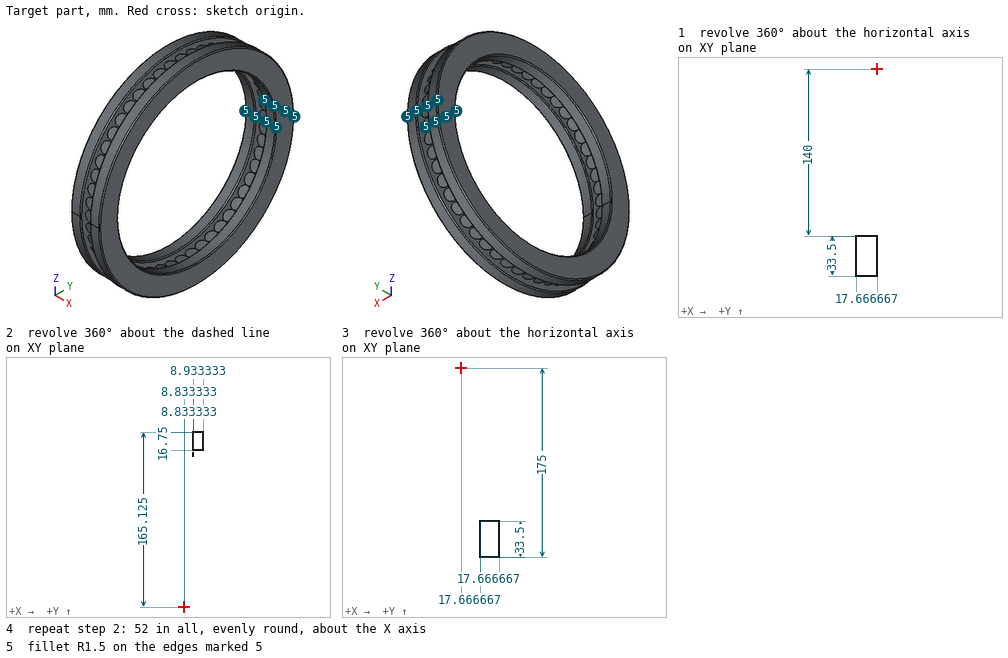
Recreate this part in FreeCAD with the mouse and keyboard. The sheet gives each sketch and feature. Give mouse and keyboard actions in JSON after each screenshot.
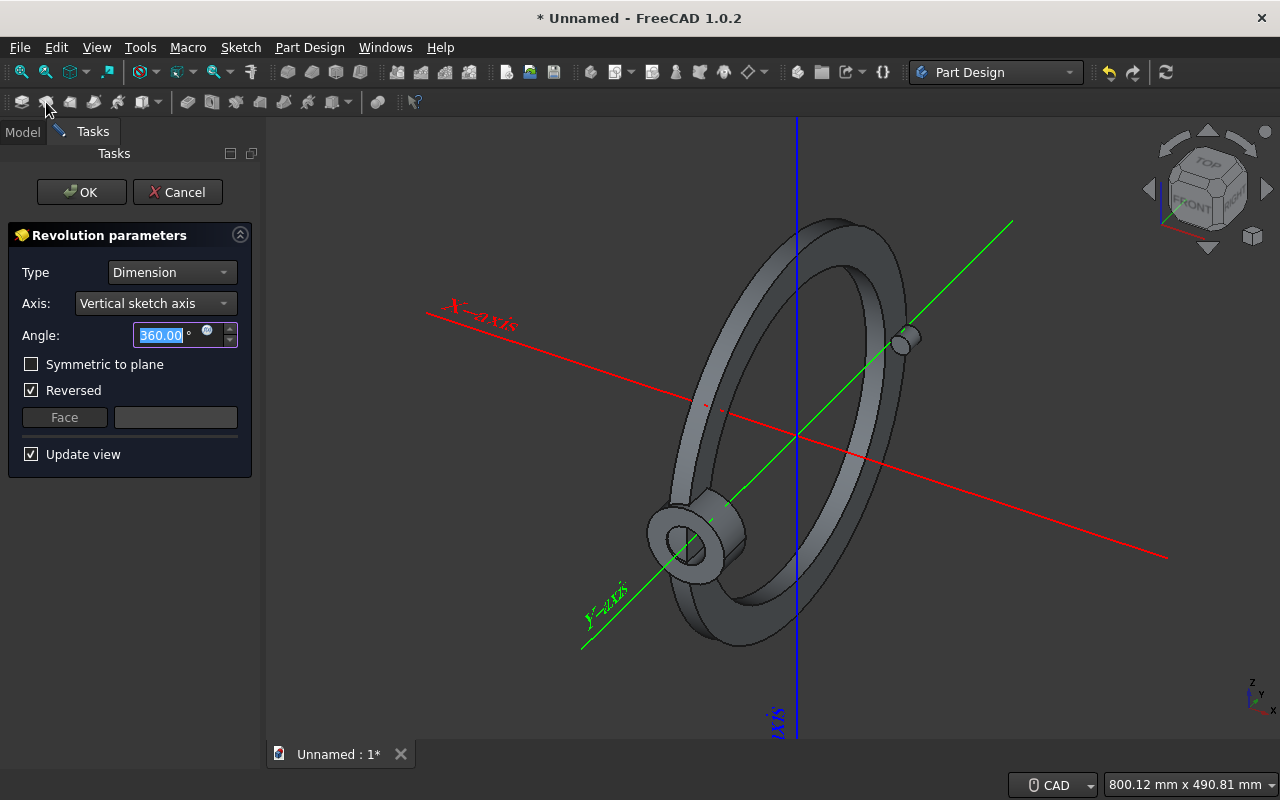
{"action": "left_click", "coordinate": [156, 304]}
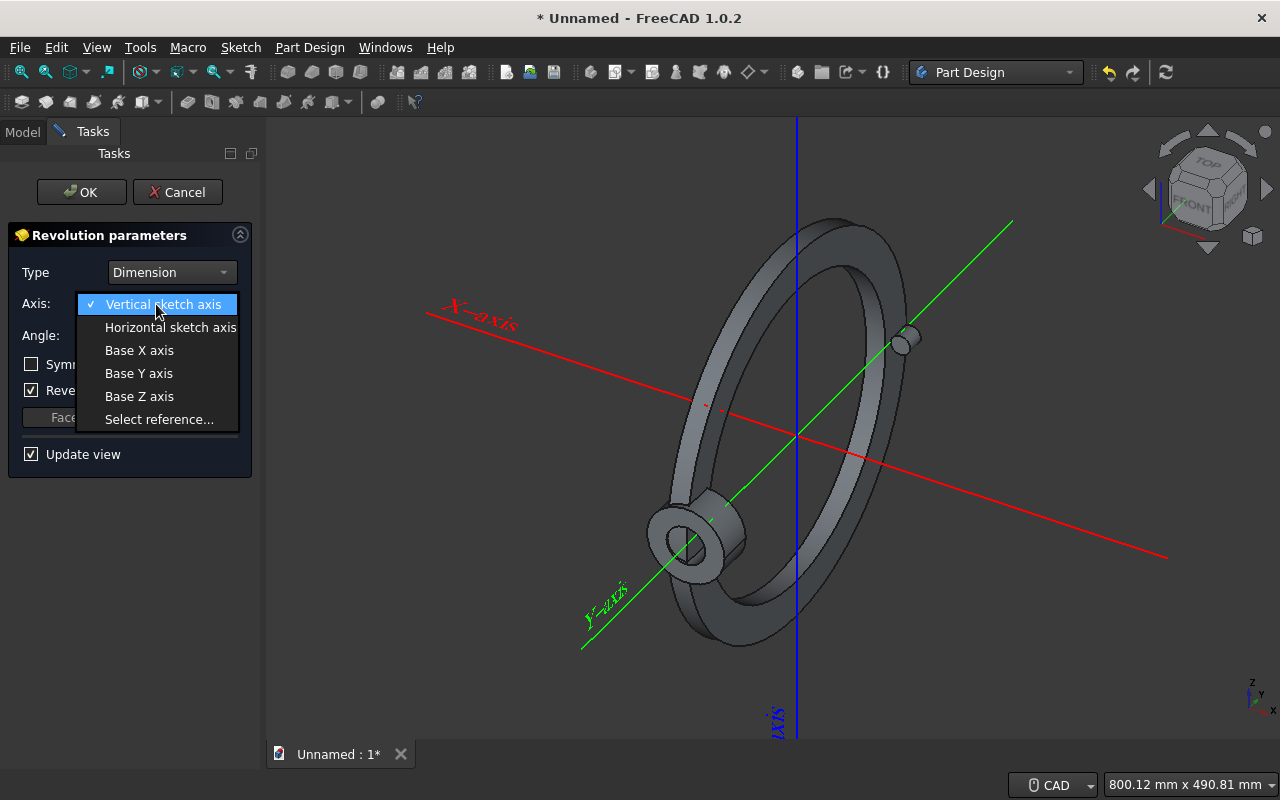
{"action": "left_click", "coordinate": [156, 328]}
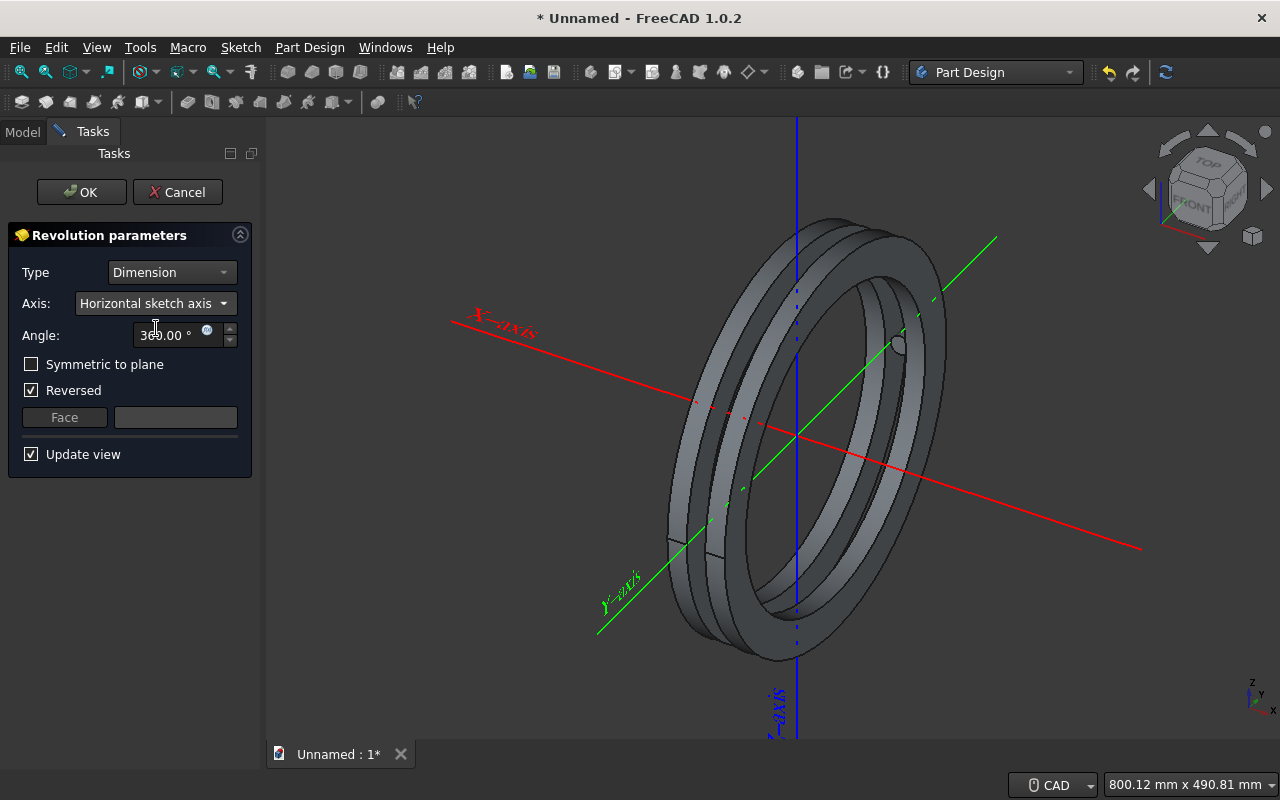
{"action": "left_click", "coordinate": [82, 192]}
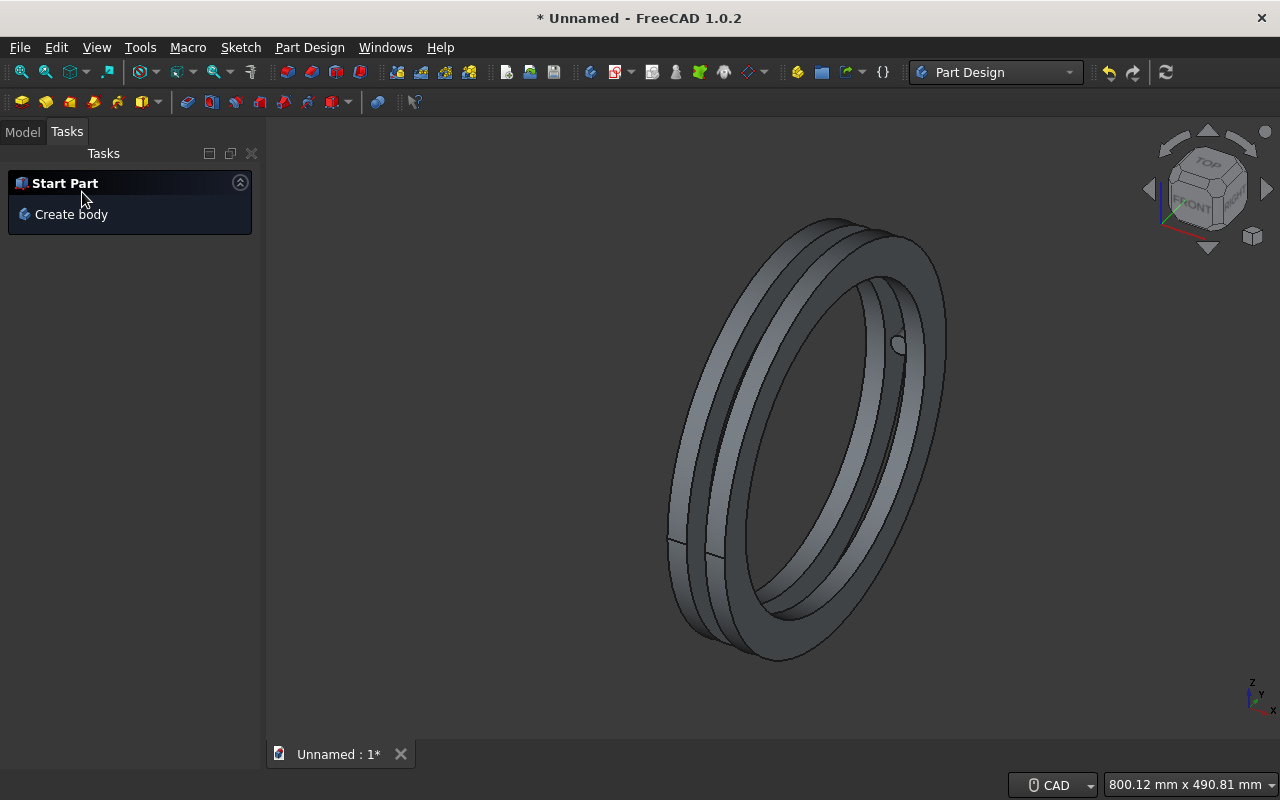
{"action": "left_click", "coordinate": [23, 131]}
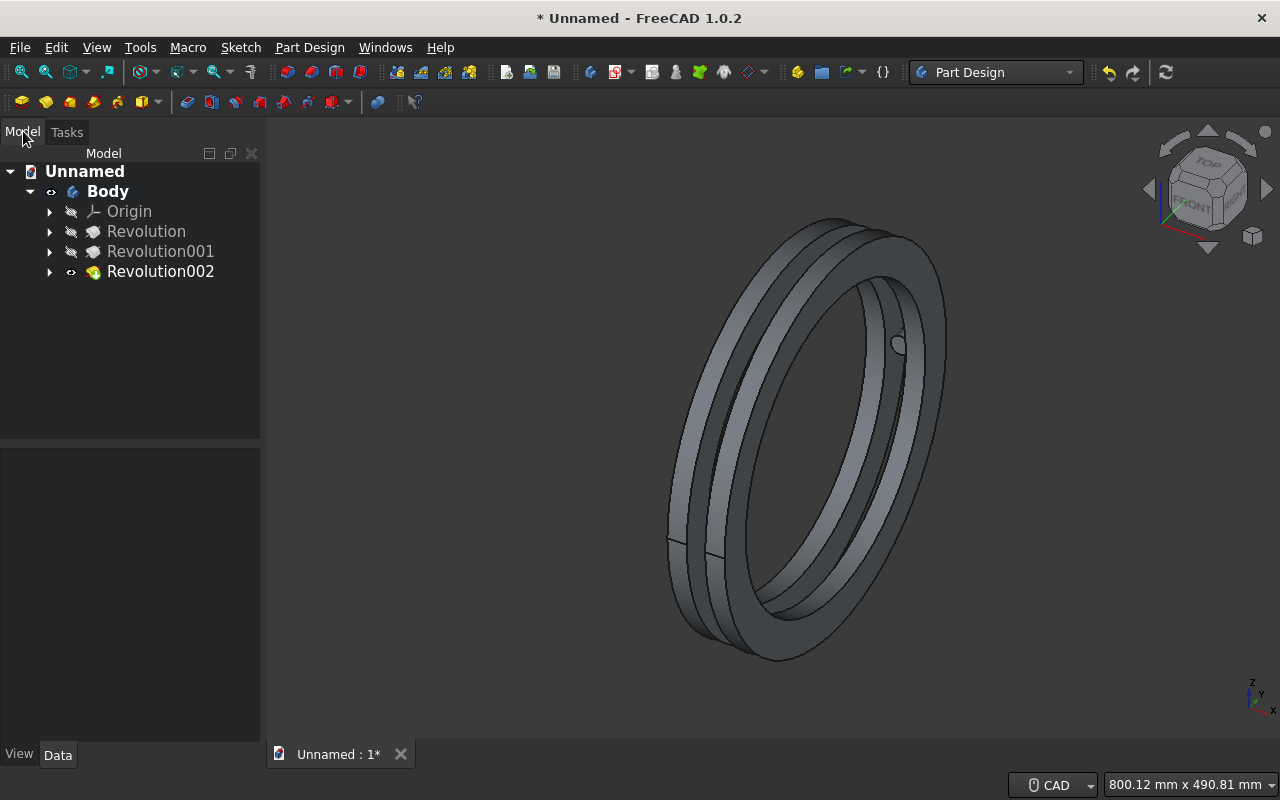
{"action": "left_click", "coordinate": [116, 252]}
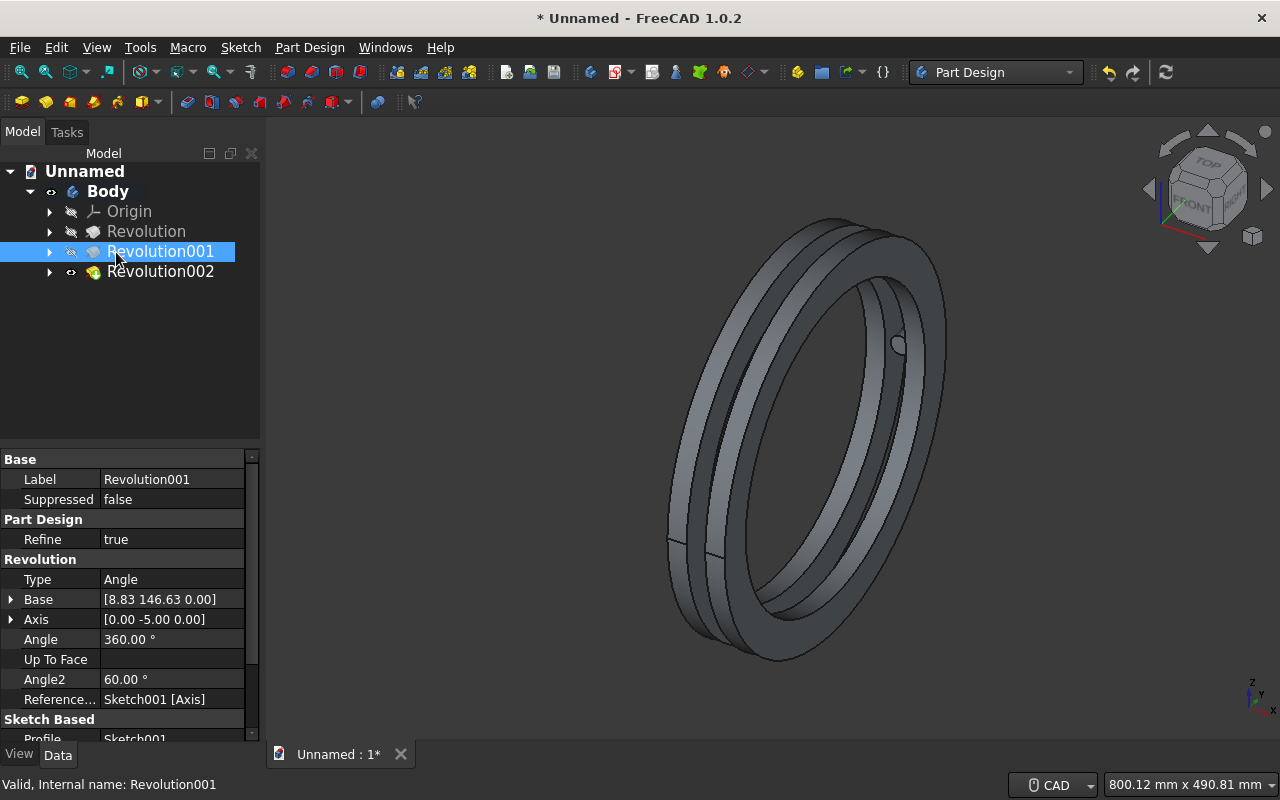
{"action": "left_click", "coordinate": [446, 72]}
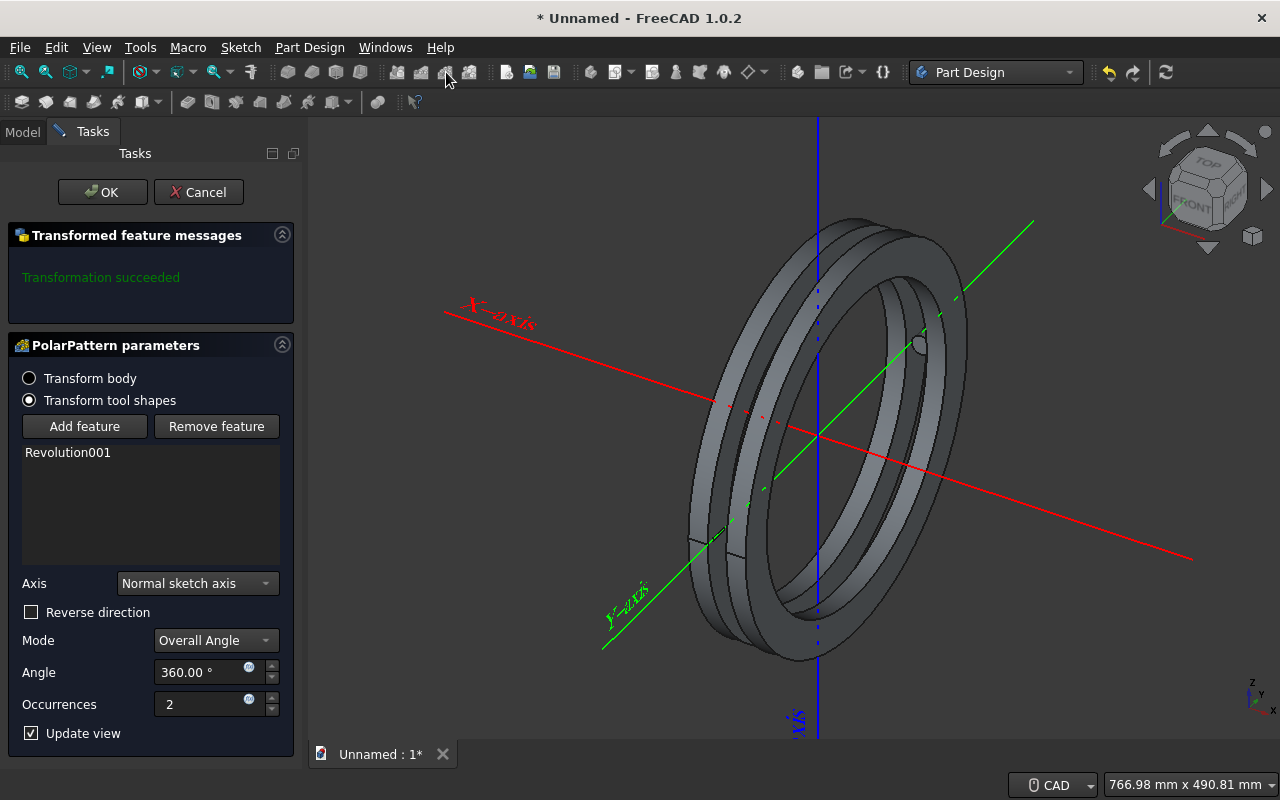
{"action": "left_click", "coordinate": [198, 584]}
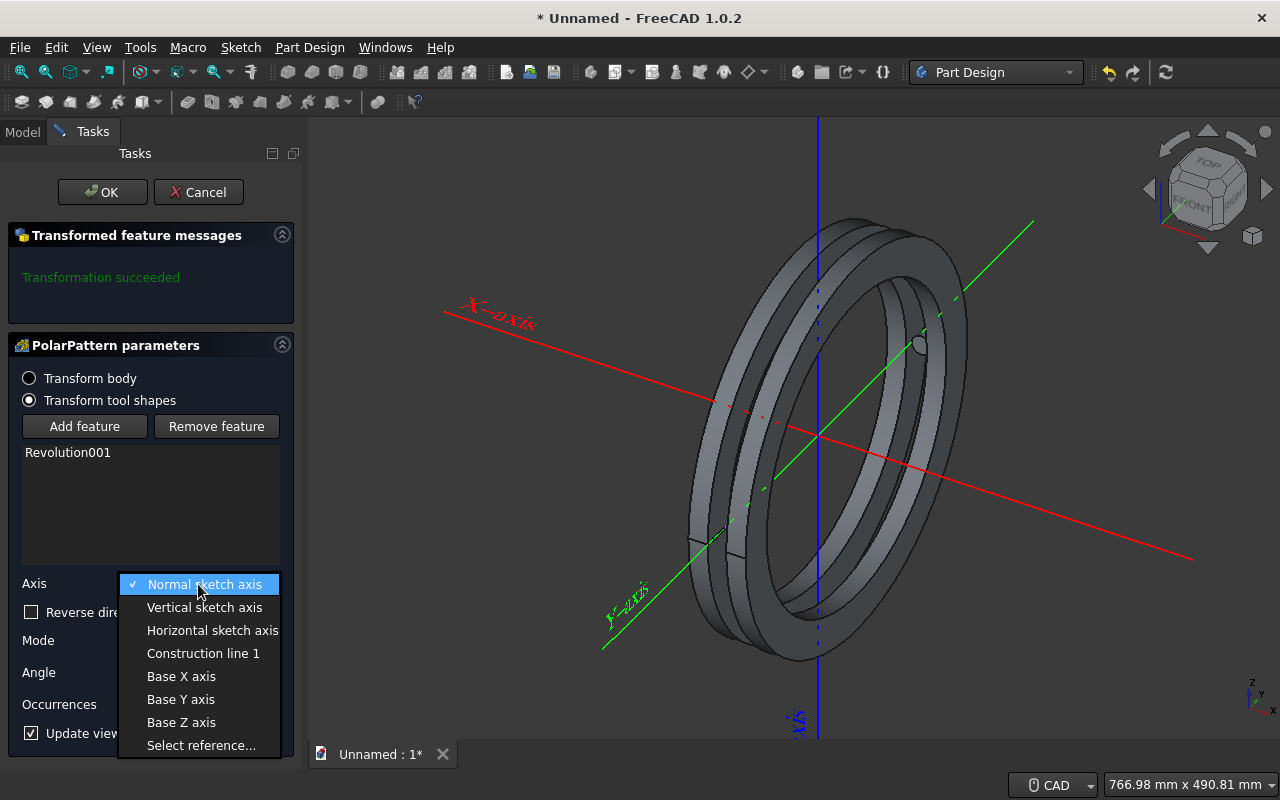
{"action": "left_click", "coordinate": [198, 676]}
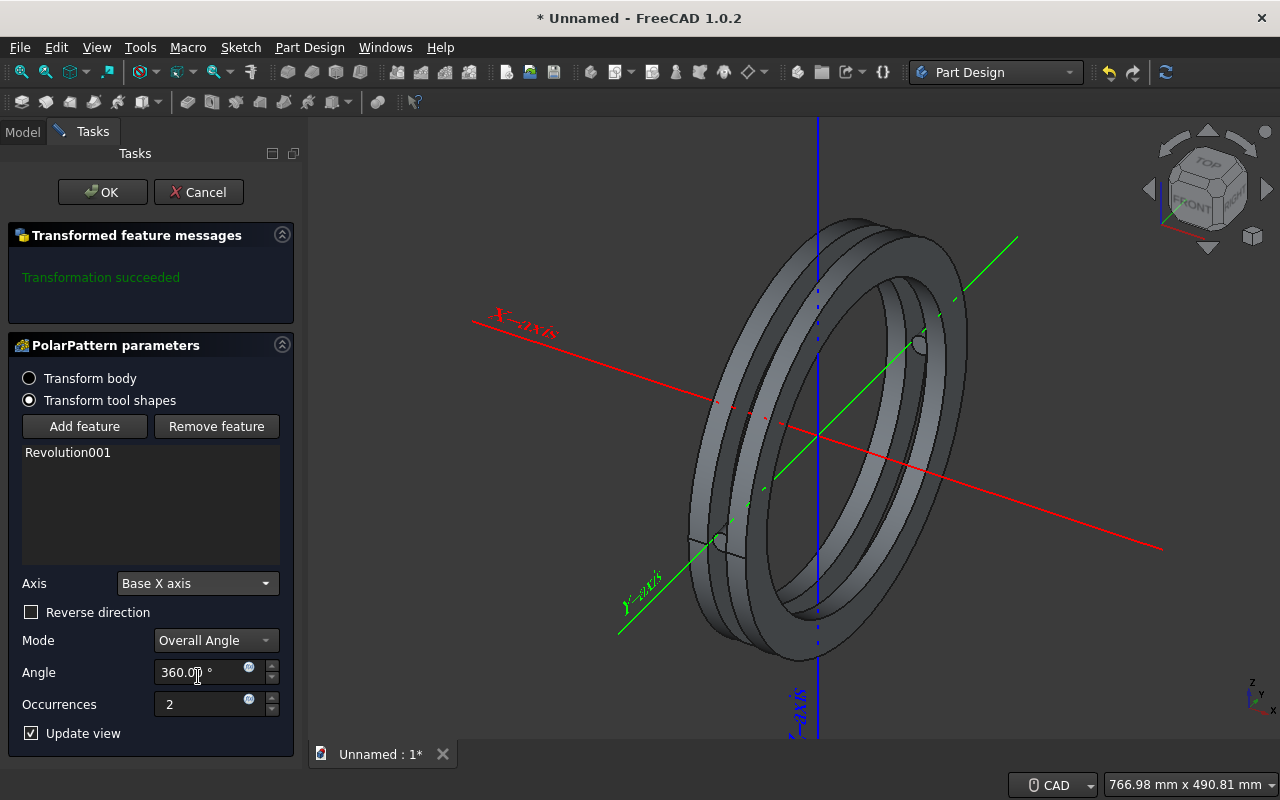
{"action": "triple_click", "coordinate": [209, 704]}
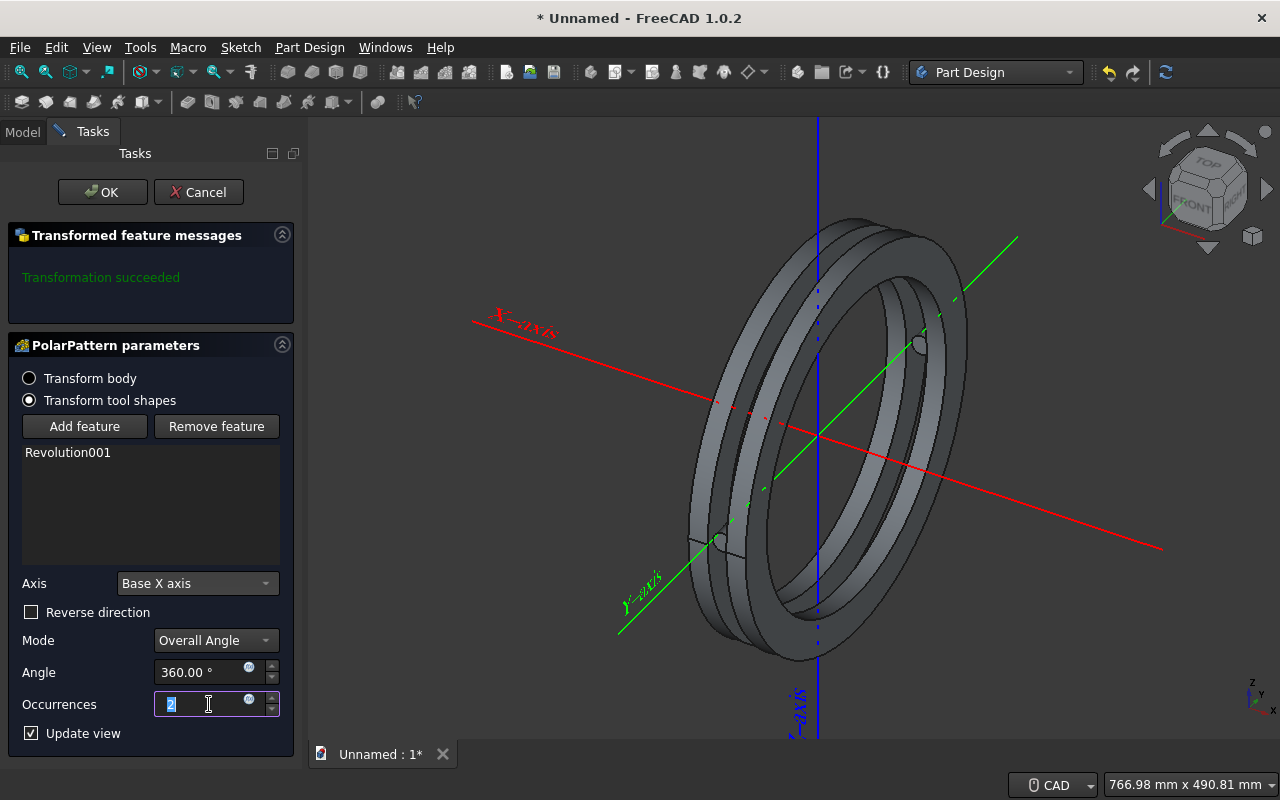
{"action": "type", "text": "52"}
{"action": "key", "text": "Tab"}